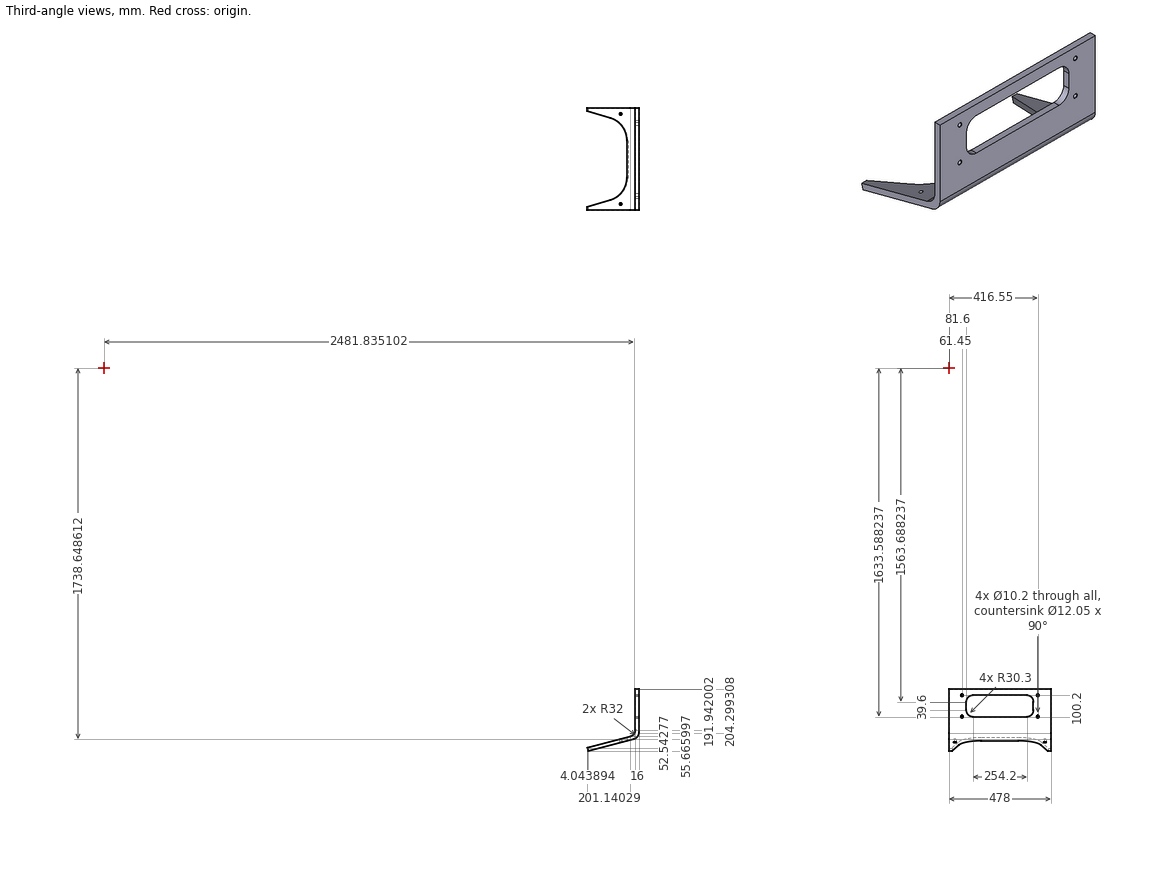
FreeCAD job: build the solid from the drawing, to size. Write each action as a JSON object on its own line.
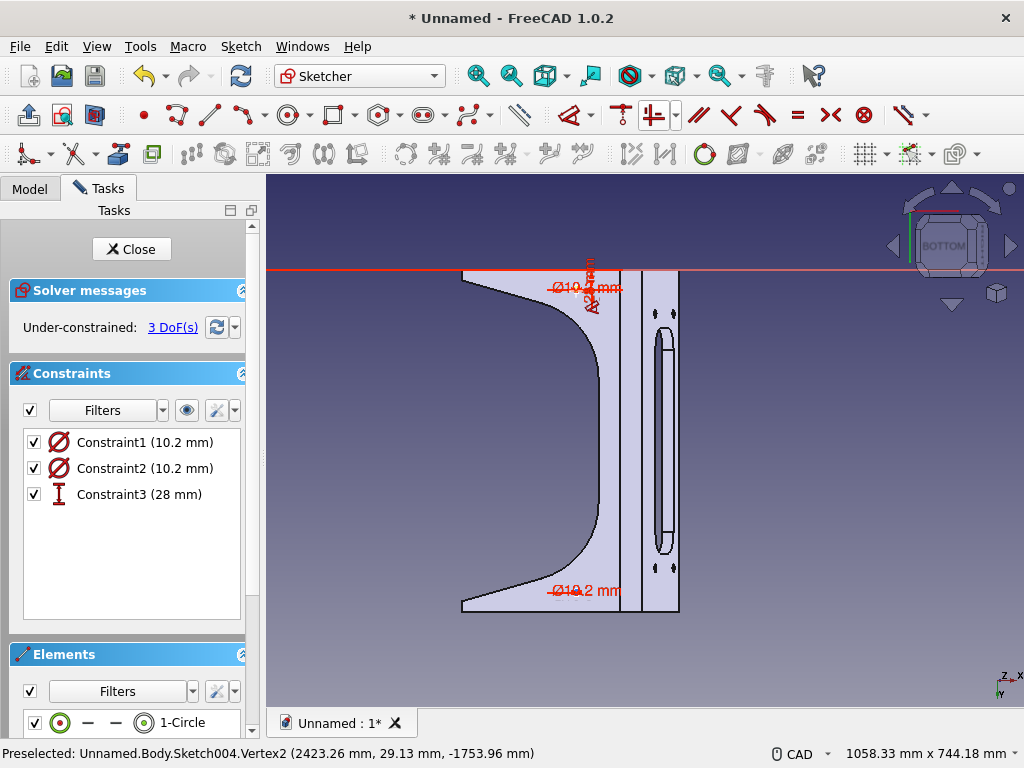
{"action": "left_click", "coordinate": [576, 593]}
{"action": "left_click", "coordinate": [610, 431]}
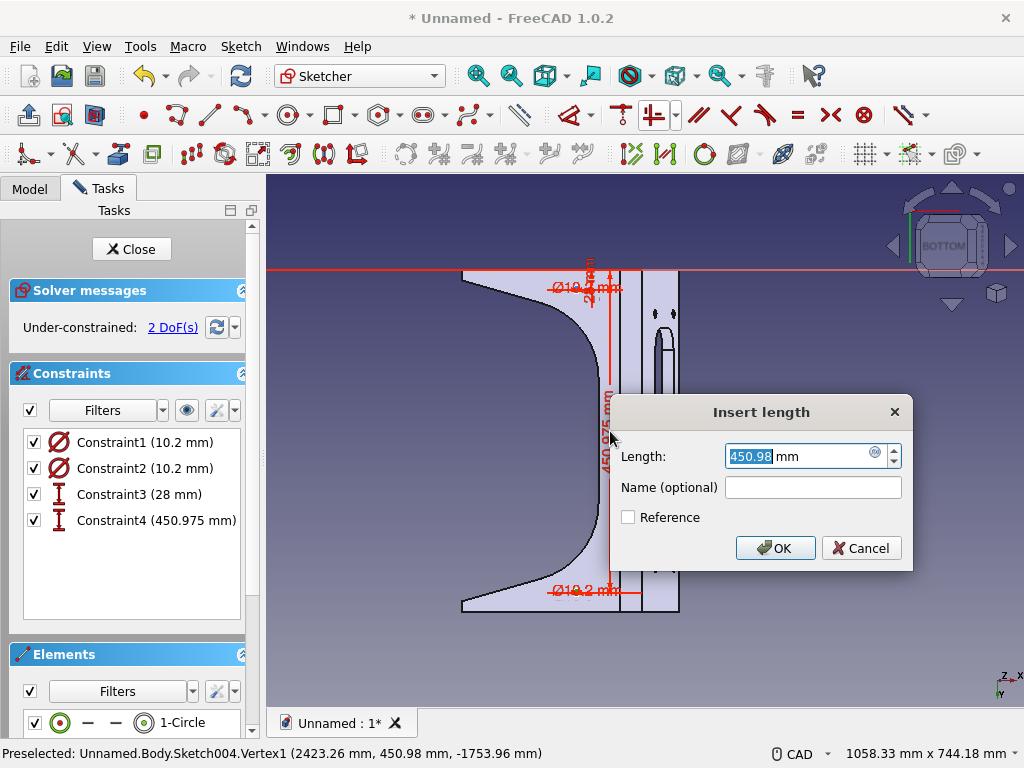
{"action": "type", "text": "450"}
{"action": "key", "text": "Return"}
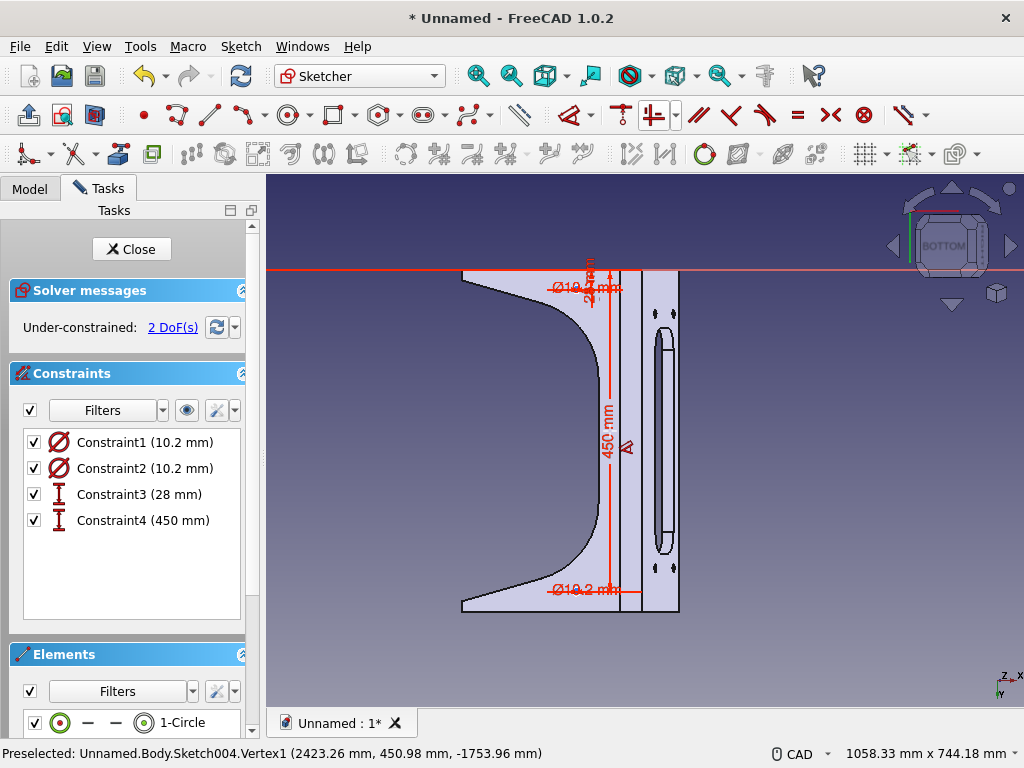
{"action": "left_click", "coordinate": [576, 592]}
{"action": "left_click", "coordinate": [435, 236]}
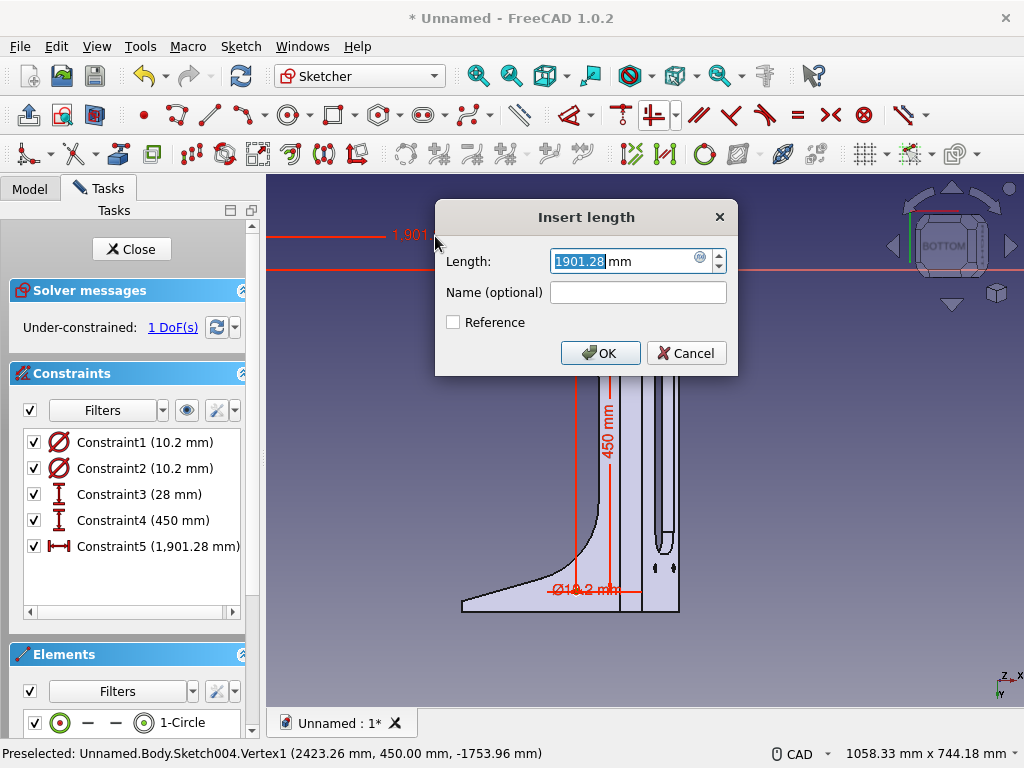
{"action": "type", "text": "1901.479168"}
{"action": "key", "text": "Return"}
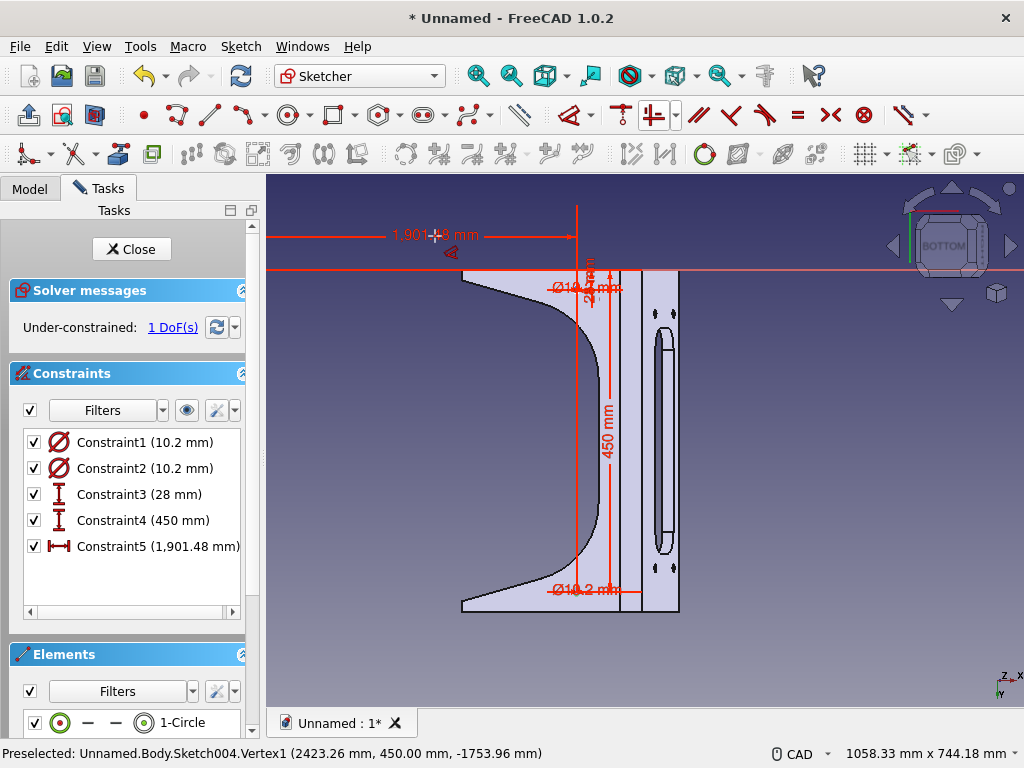
{"action": "left_click", "coordinate": [576, 290]}
{"action": "left_click", "coordinate": [336, 236]}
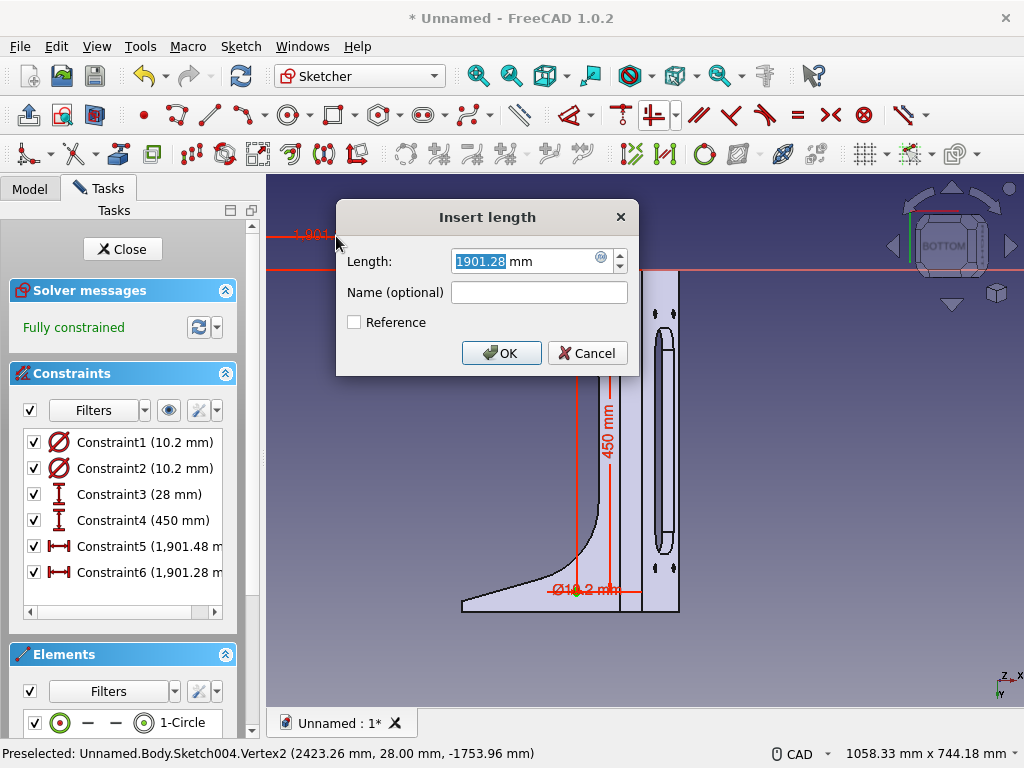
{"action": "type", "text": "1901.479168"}
{"action": "key", "text": "Return"}
{"action": "key", "text": "Escape"}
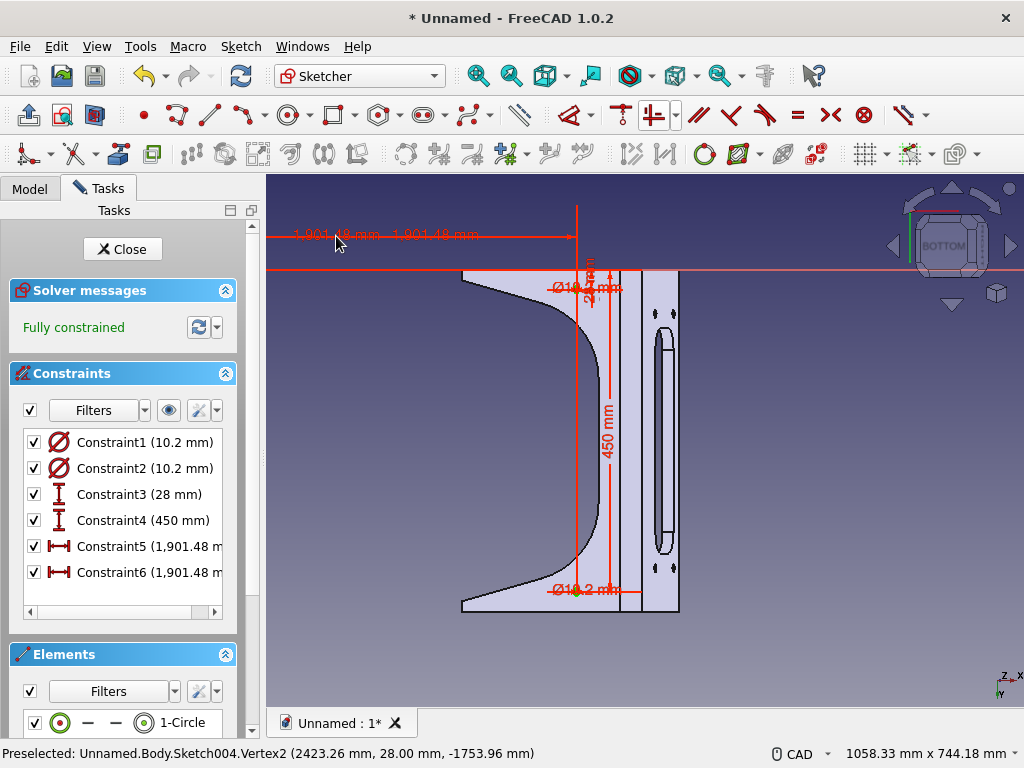
{"action": "left_click", "coordinate": [123, 249]}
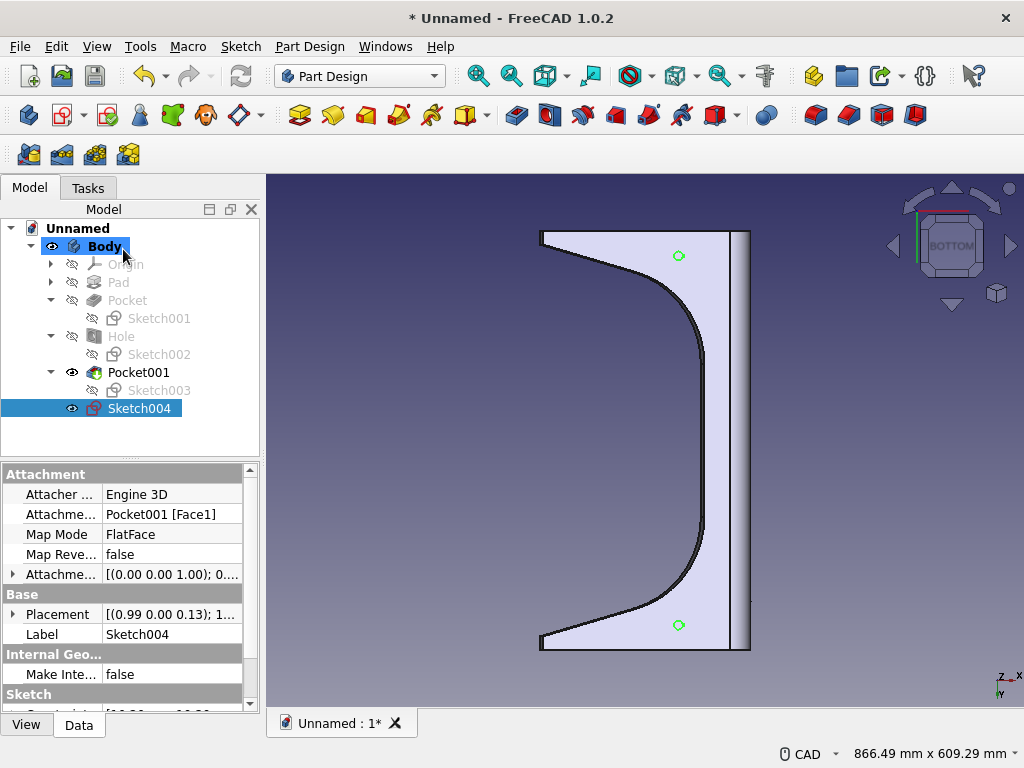
{"action": "left_click", "coordinate": [550, 116]}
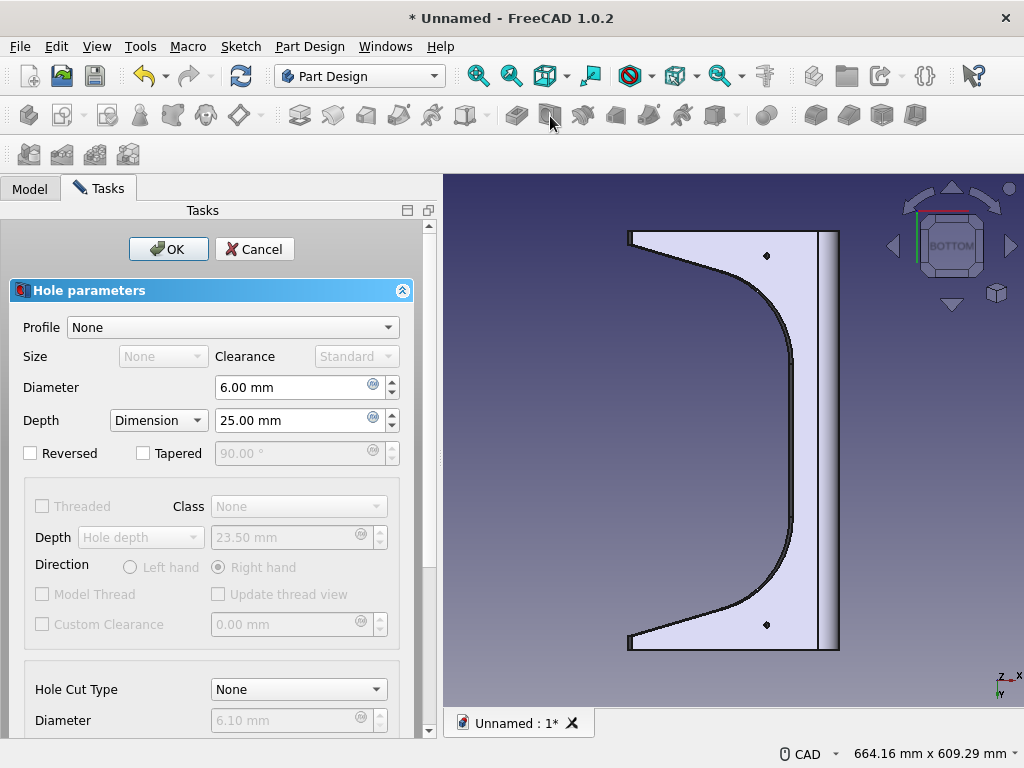
{"action": "triple_click", "coordinate": [300, 388]}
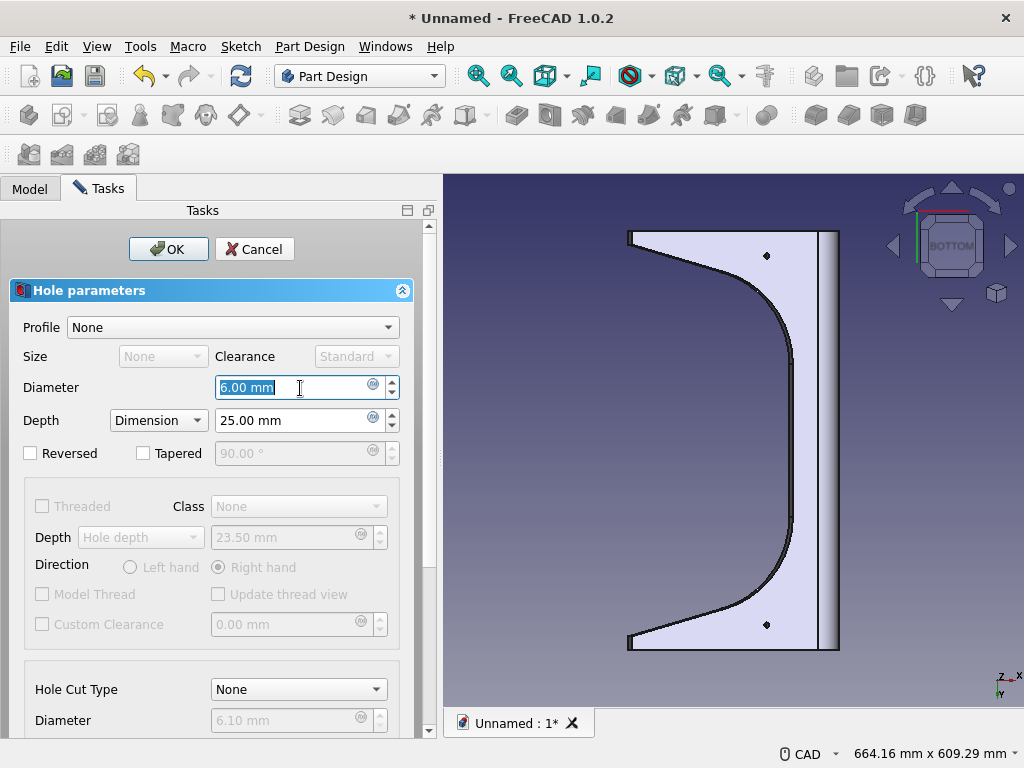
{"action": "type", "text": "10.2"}
{"action": "key", "text": "Tab"}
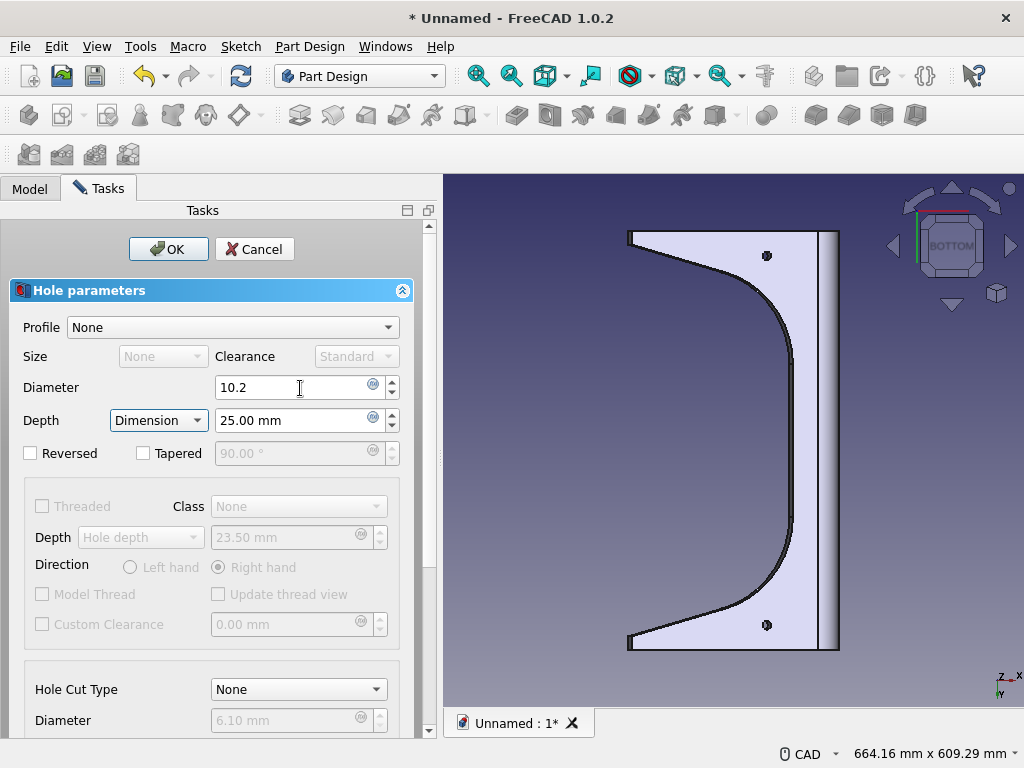
{"action": "left_click", "coordinate": [160, 420]}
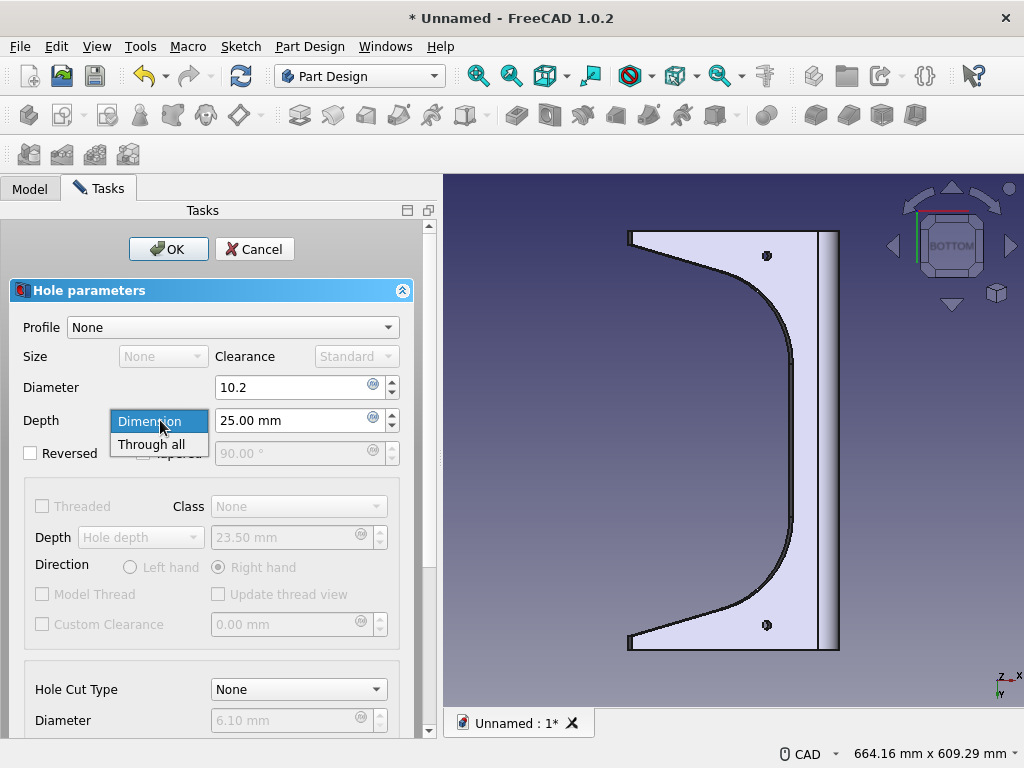
{"action": "left_click", "coordinate": [158, 444]}